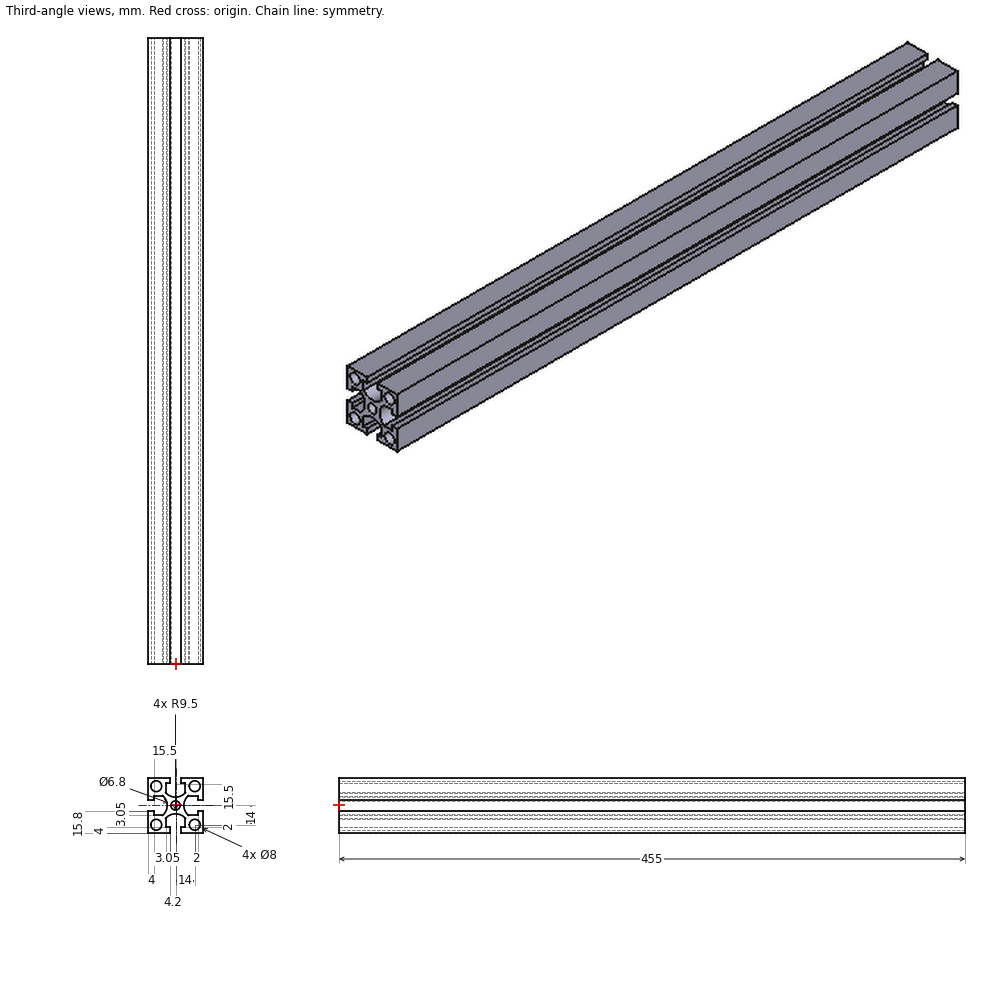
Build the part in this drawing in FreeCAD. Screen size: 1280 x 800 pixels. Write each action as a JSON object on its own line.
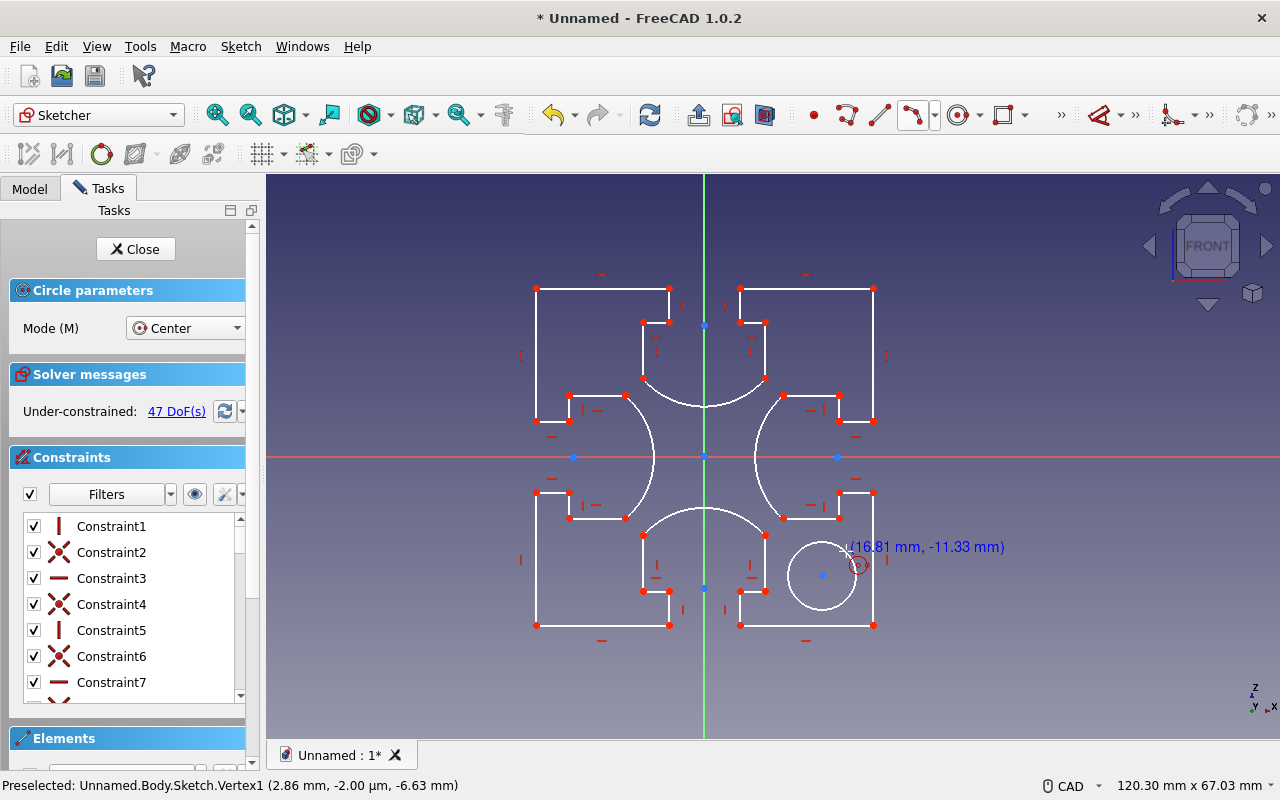
{"action": "left_click", "coordinate": [704, 456]}
{"action": "left_click", "coordinate": [725, 436]}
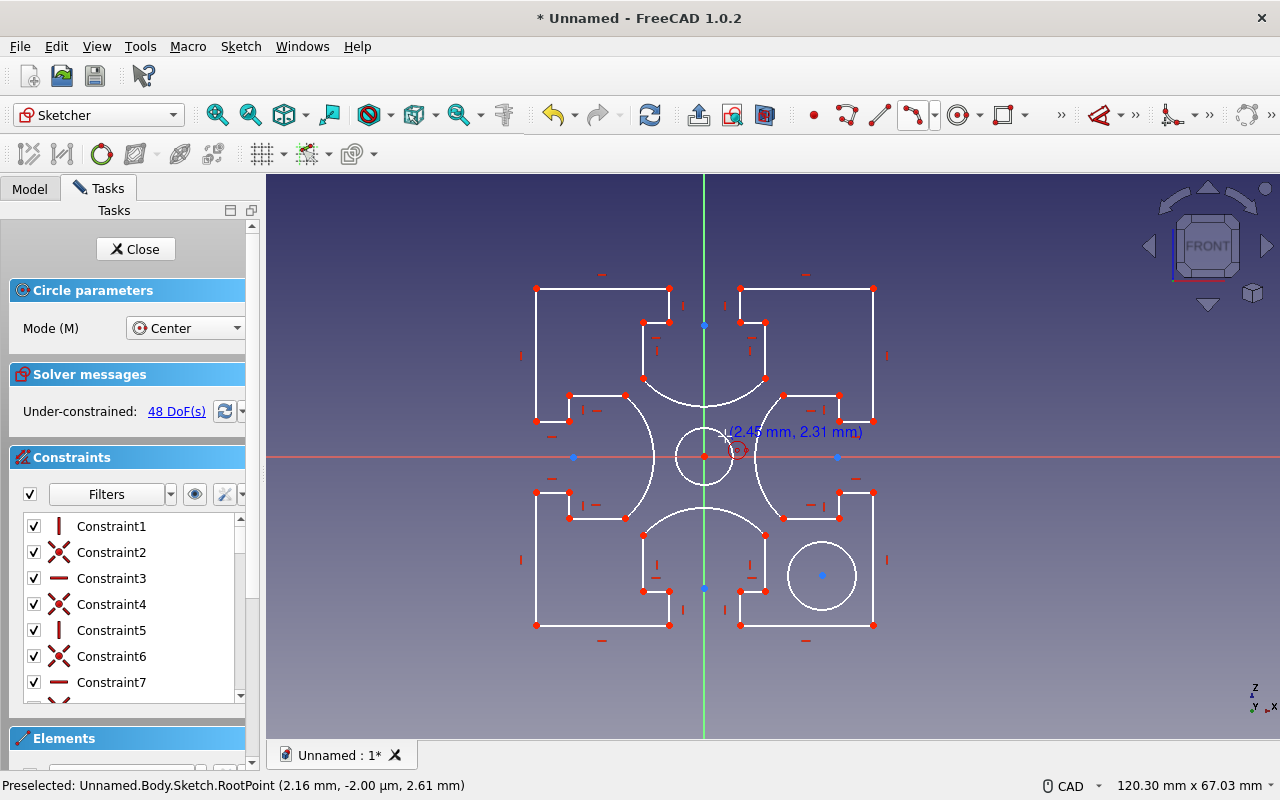
{"action": "left_click", "coordinate": [586, 575]}
{"action": "left_click", "coordinate": [610, 551]}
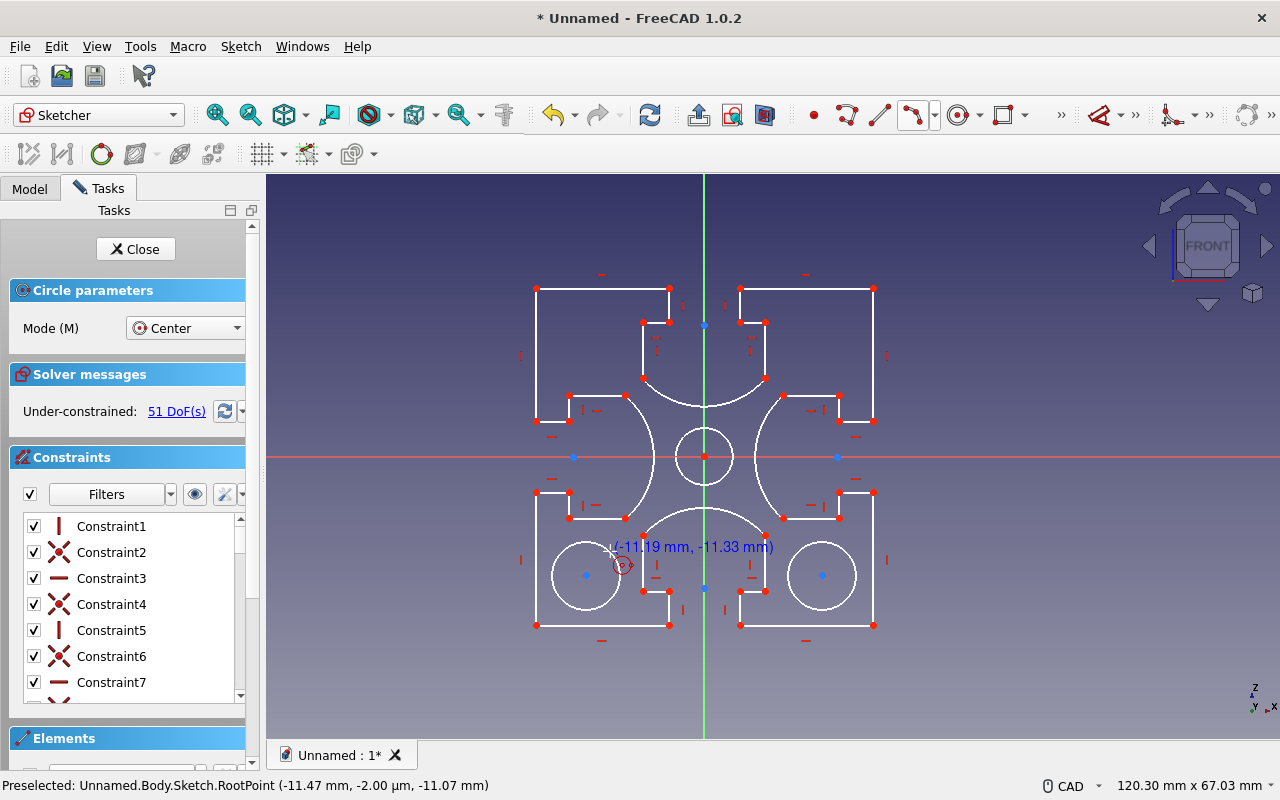
{"action": "left_click", "coordinate": [822, 338]}
{"action": "left_click", "coordinate": [846, 315]}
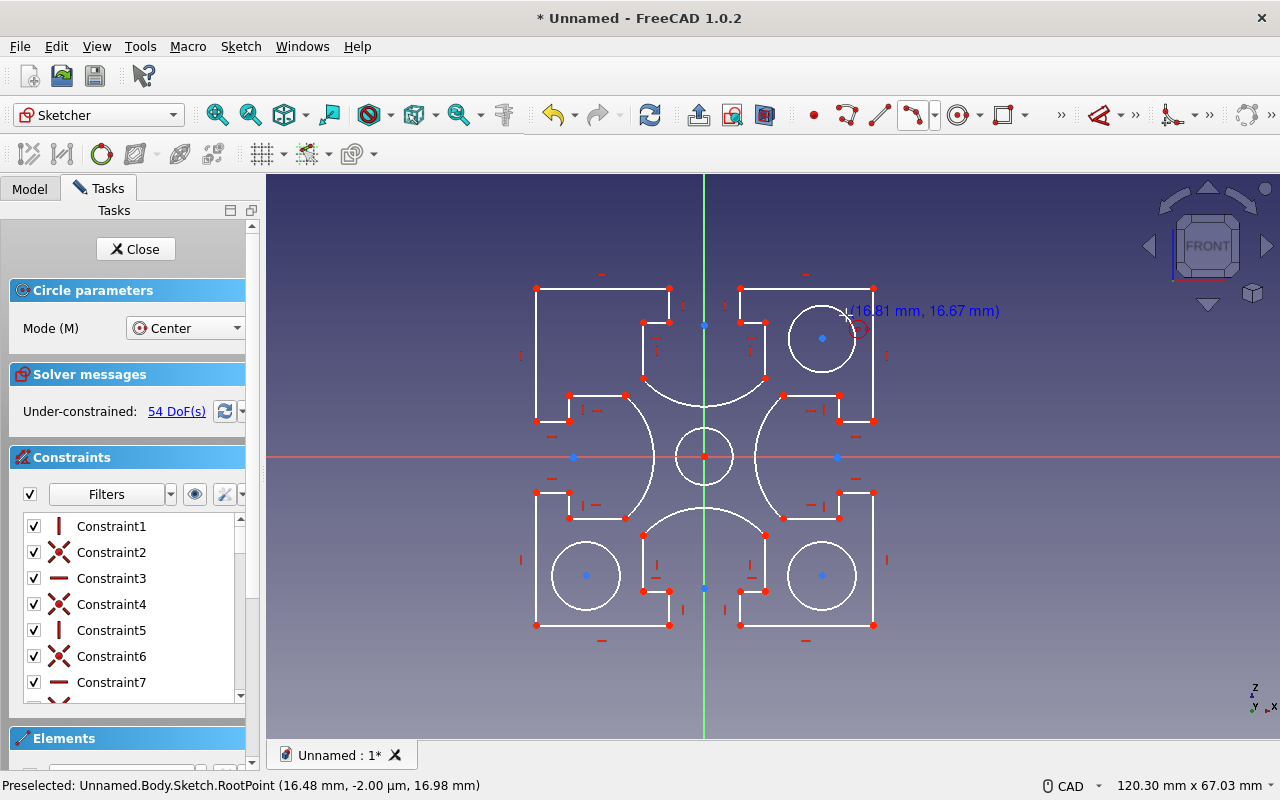
{"action": "left_click", "coordinate": [586, 338]}
{"action": "left_click", "coordinate": [610, 315]}
{"action": "key", "text": "Escape"}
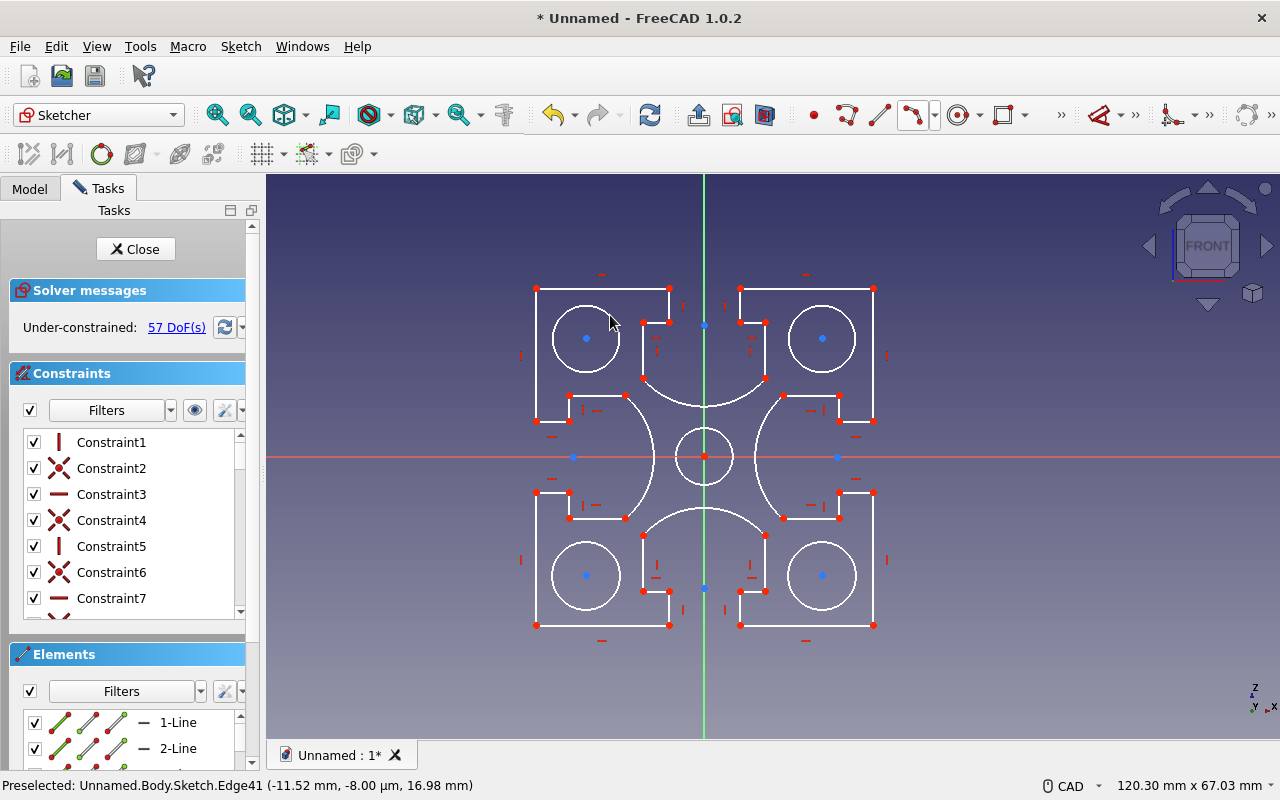
{"action": "left_click", "coordinate": [649, 485]}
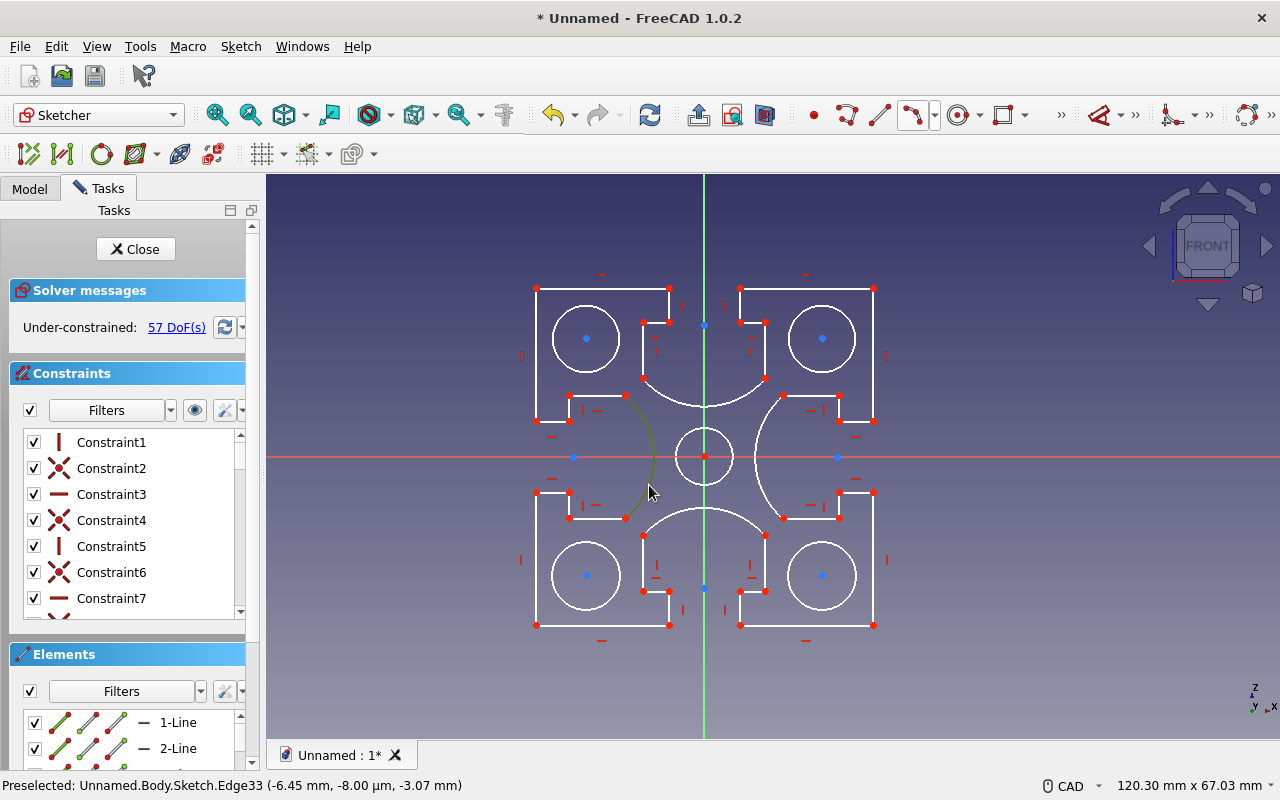
{"action": "left_click", "coordinate": [677, 402]}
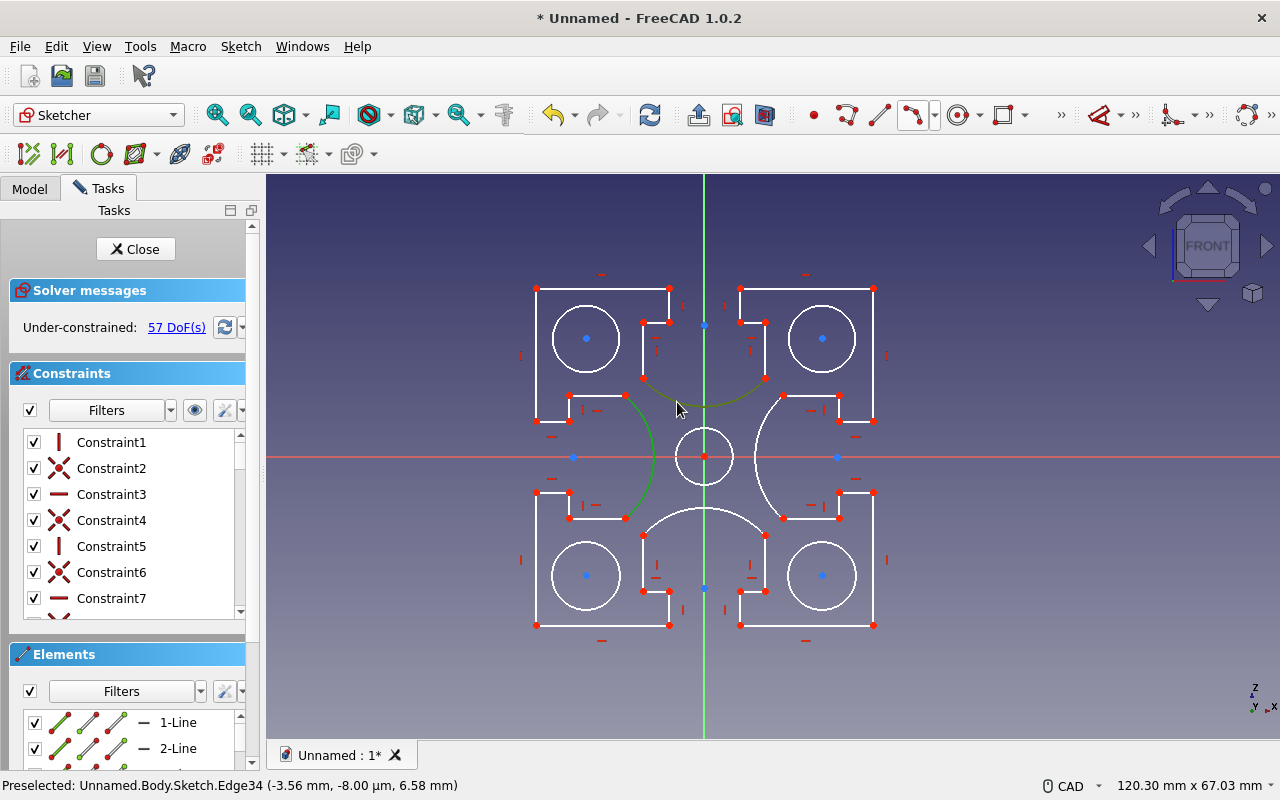
{"action": "left_click", "coordinate": [760, 430]}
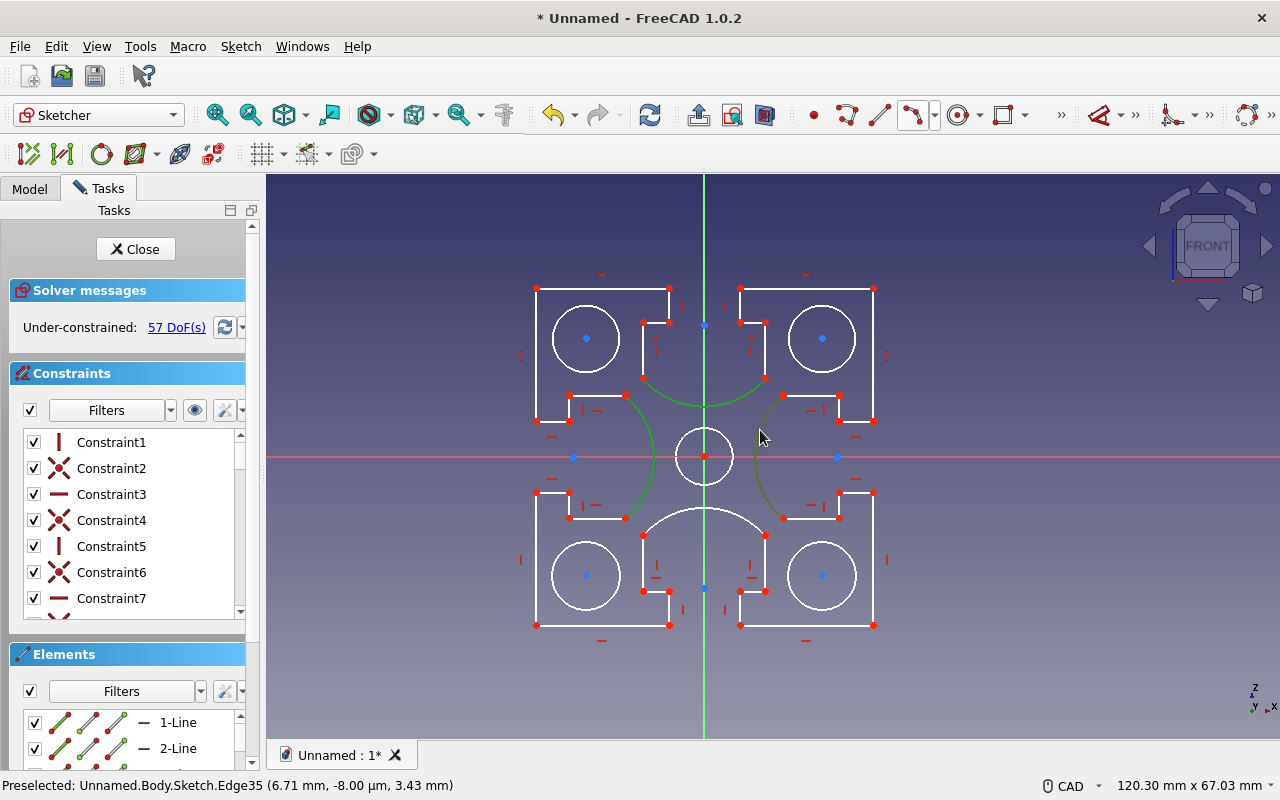
{"action": "left_click", "coordinate": [731, 513]}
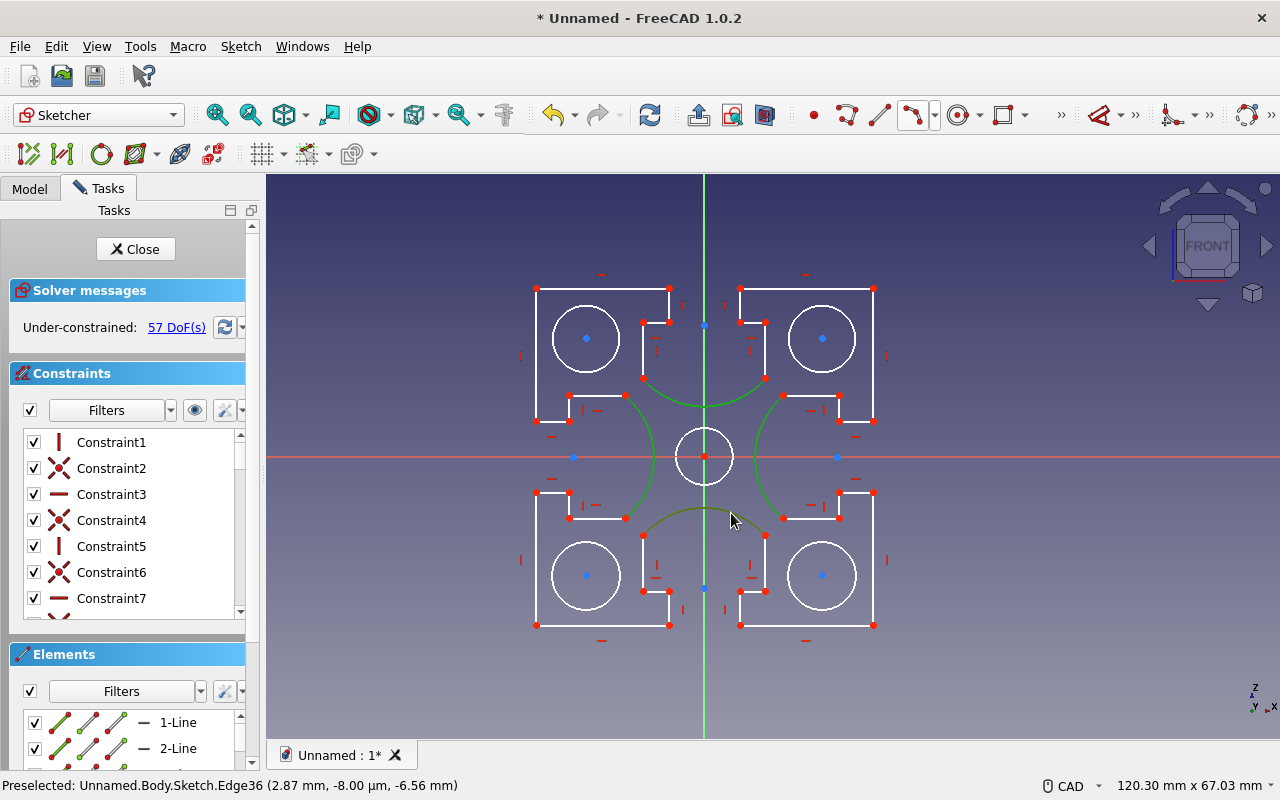
{"action": "key", "text": "e"}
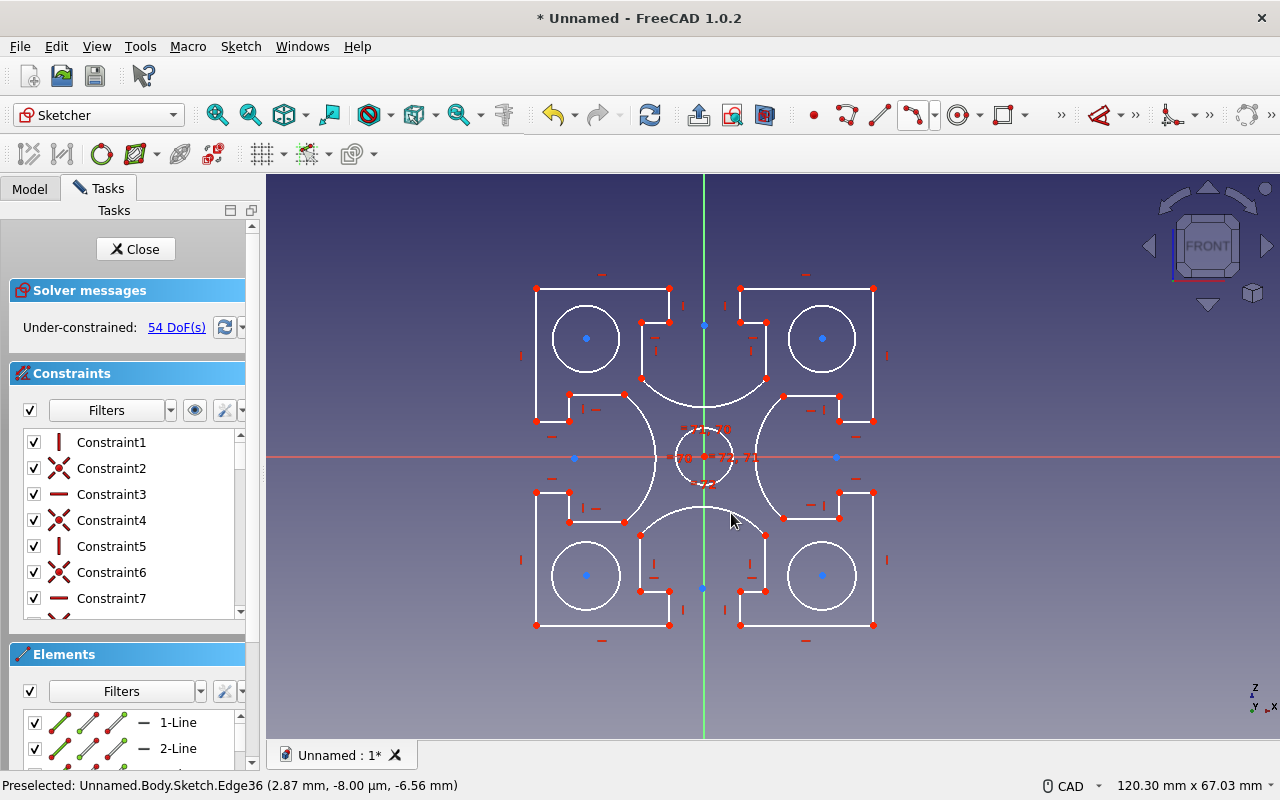
{"action": "left_click", "coordinate": [846, 552]}